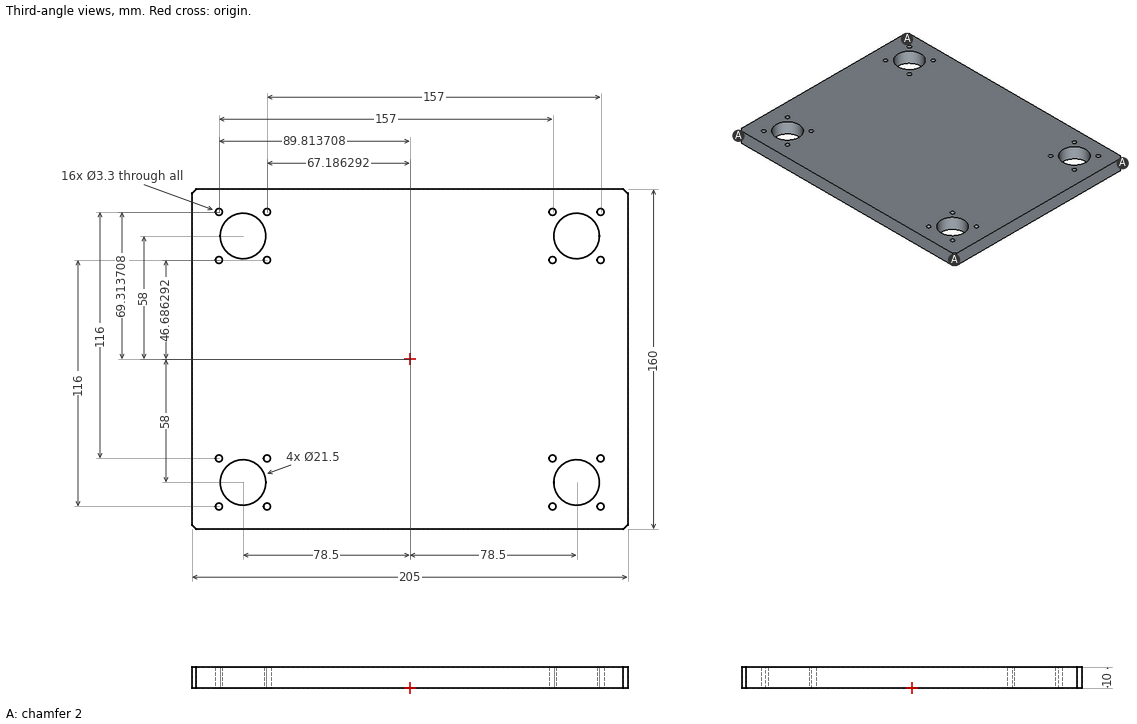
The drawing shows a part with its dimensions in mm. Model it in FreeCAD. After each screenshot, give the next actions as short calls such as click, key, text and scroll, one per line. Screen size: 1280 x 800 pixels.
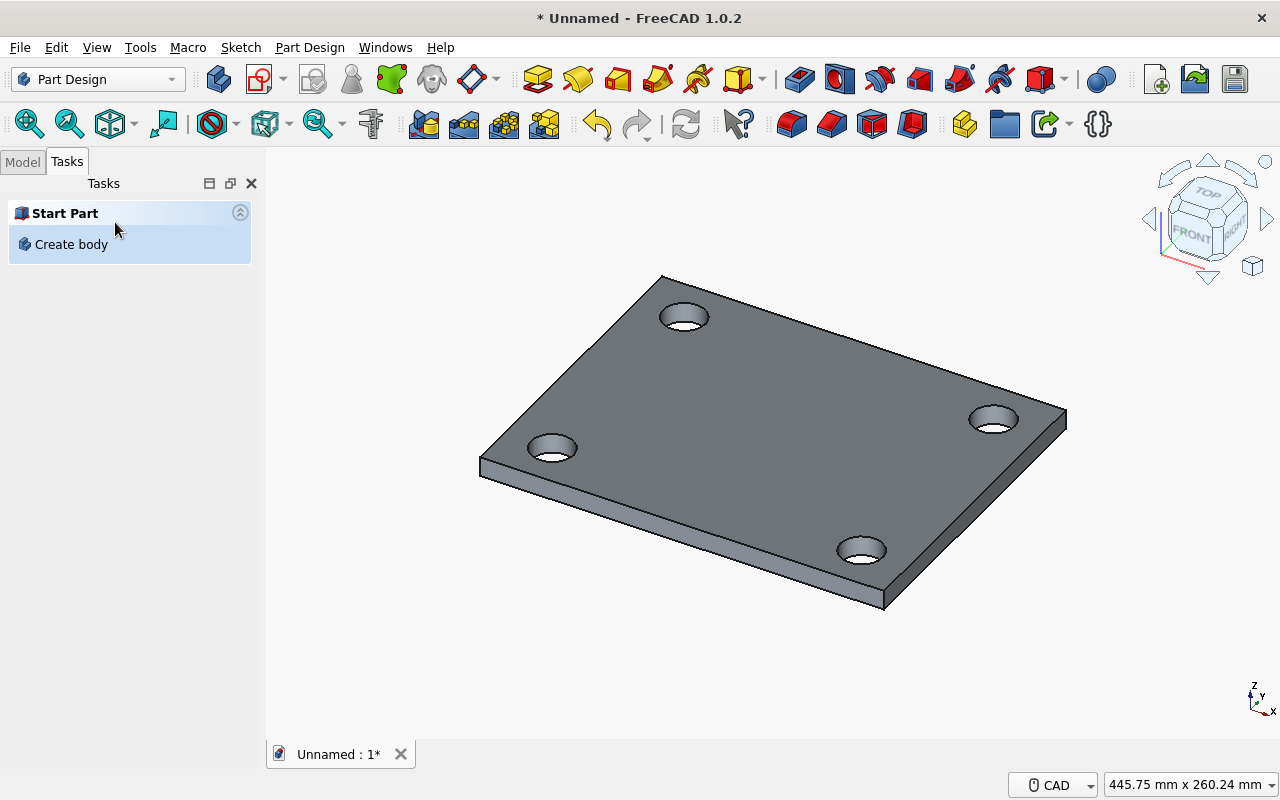
click(773, 433)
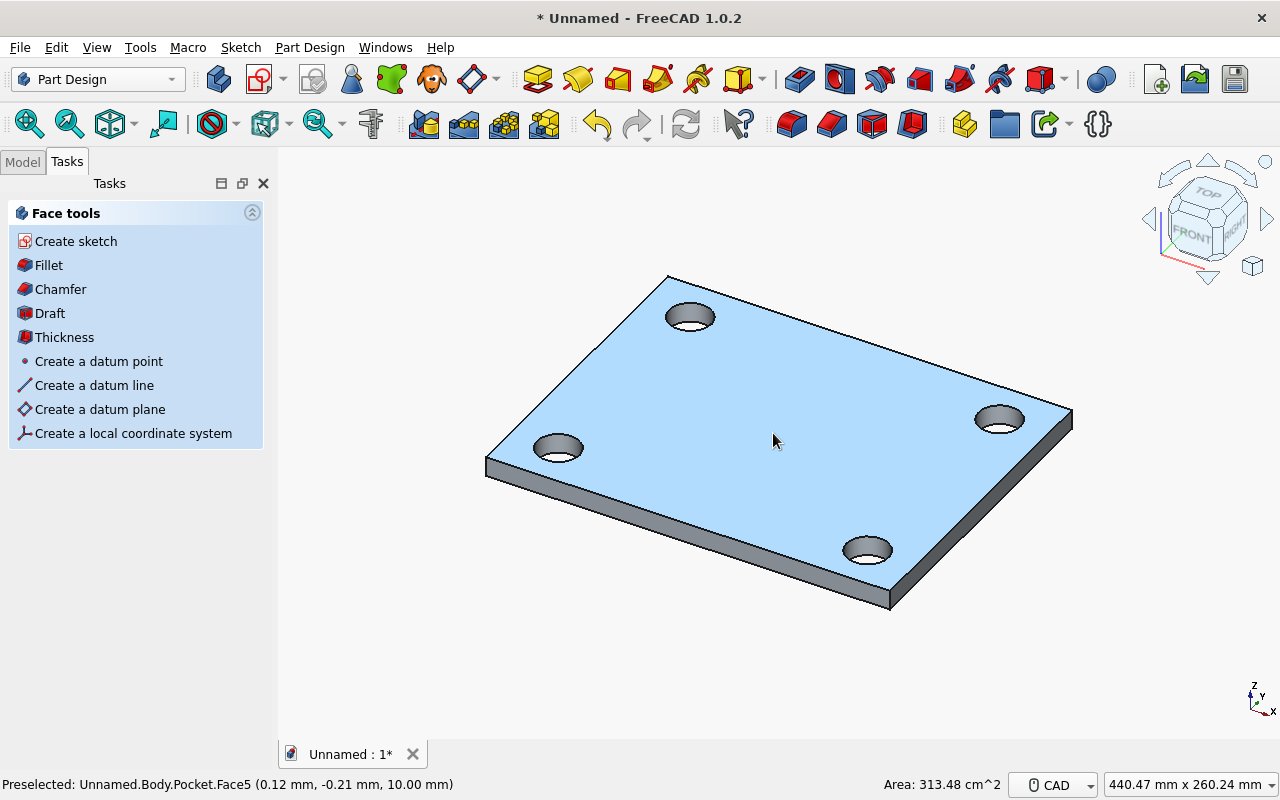
click(260, 80)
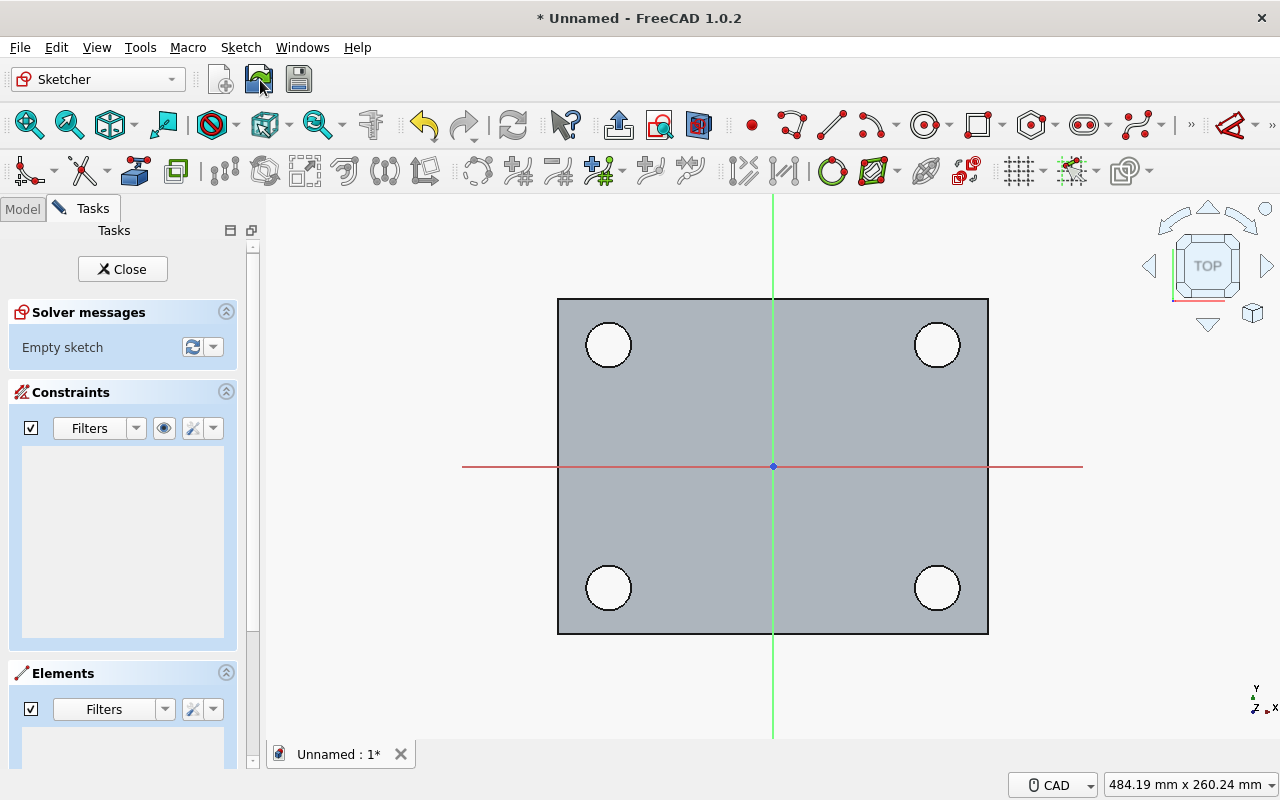
key(g)
key(c)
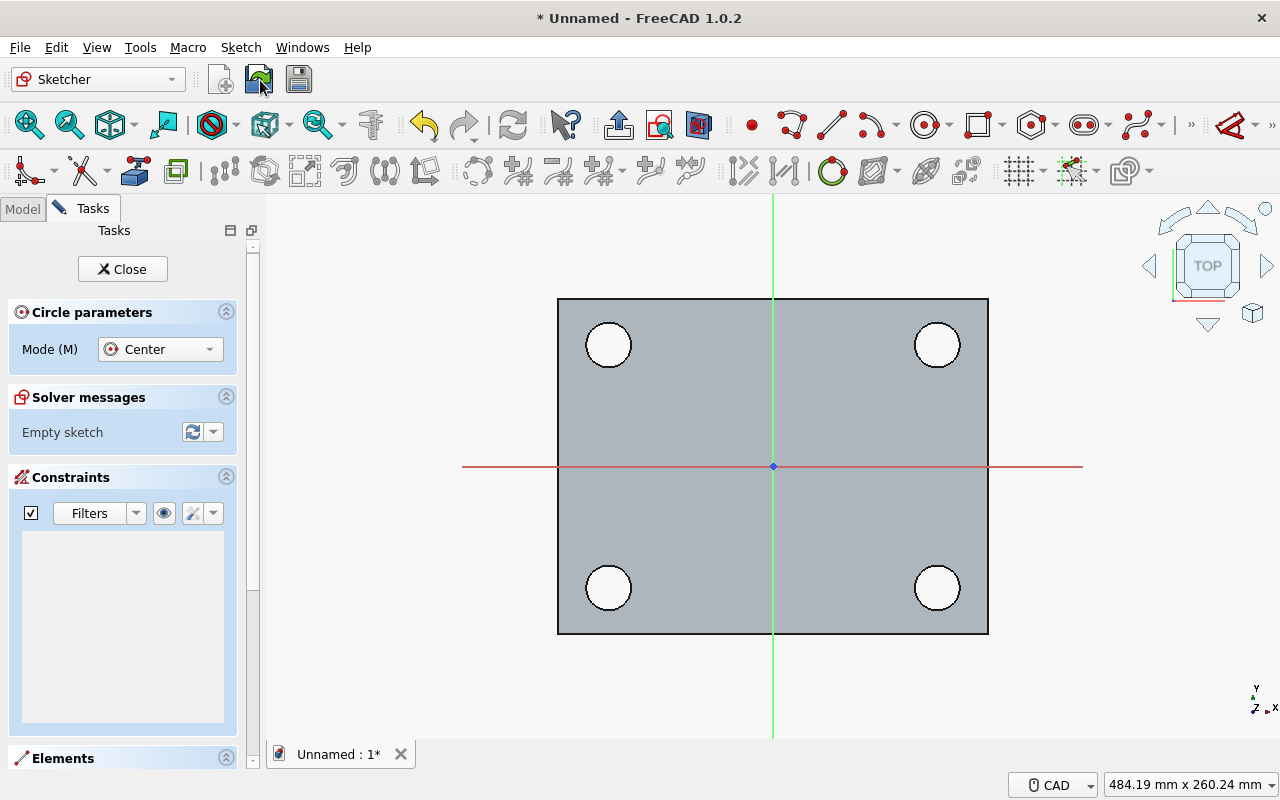
scroll(585, 321, up, 10)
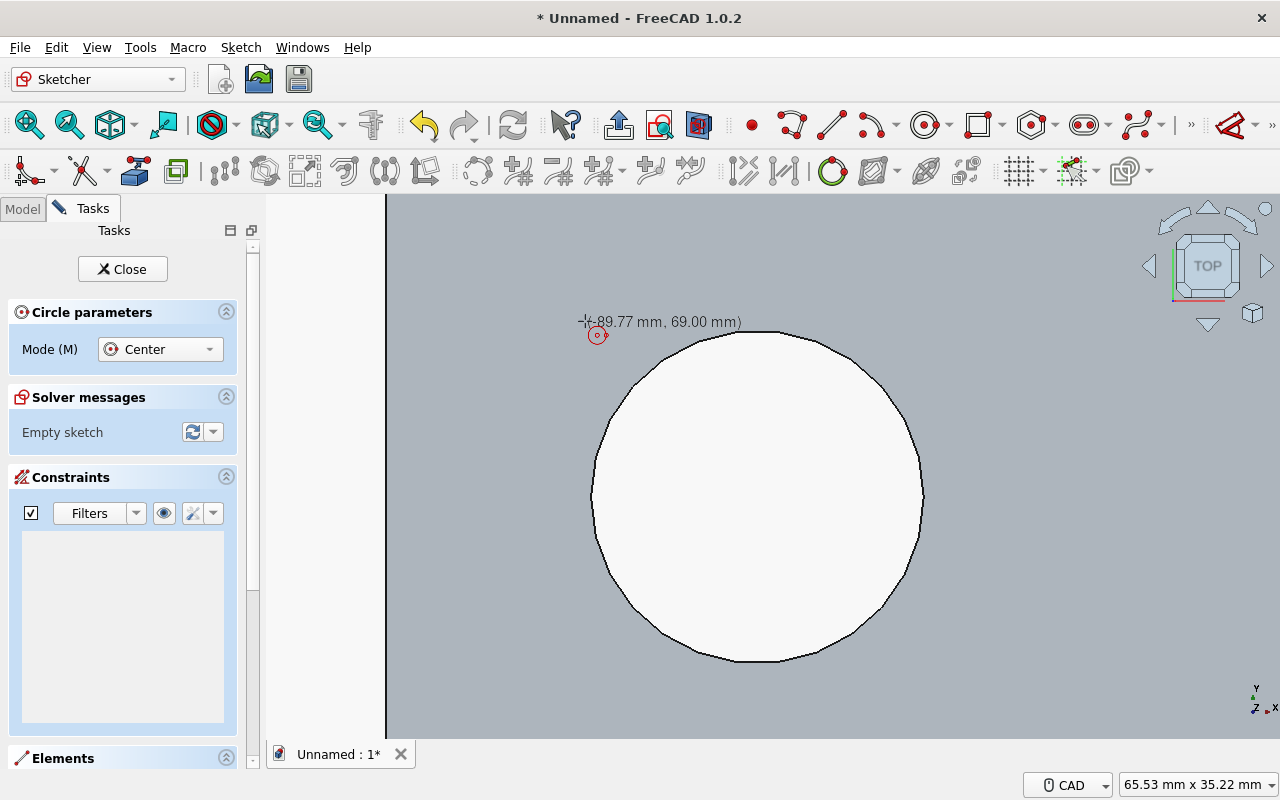
scroll(453, 283, down, 9)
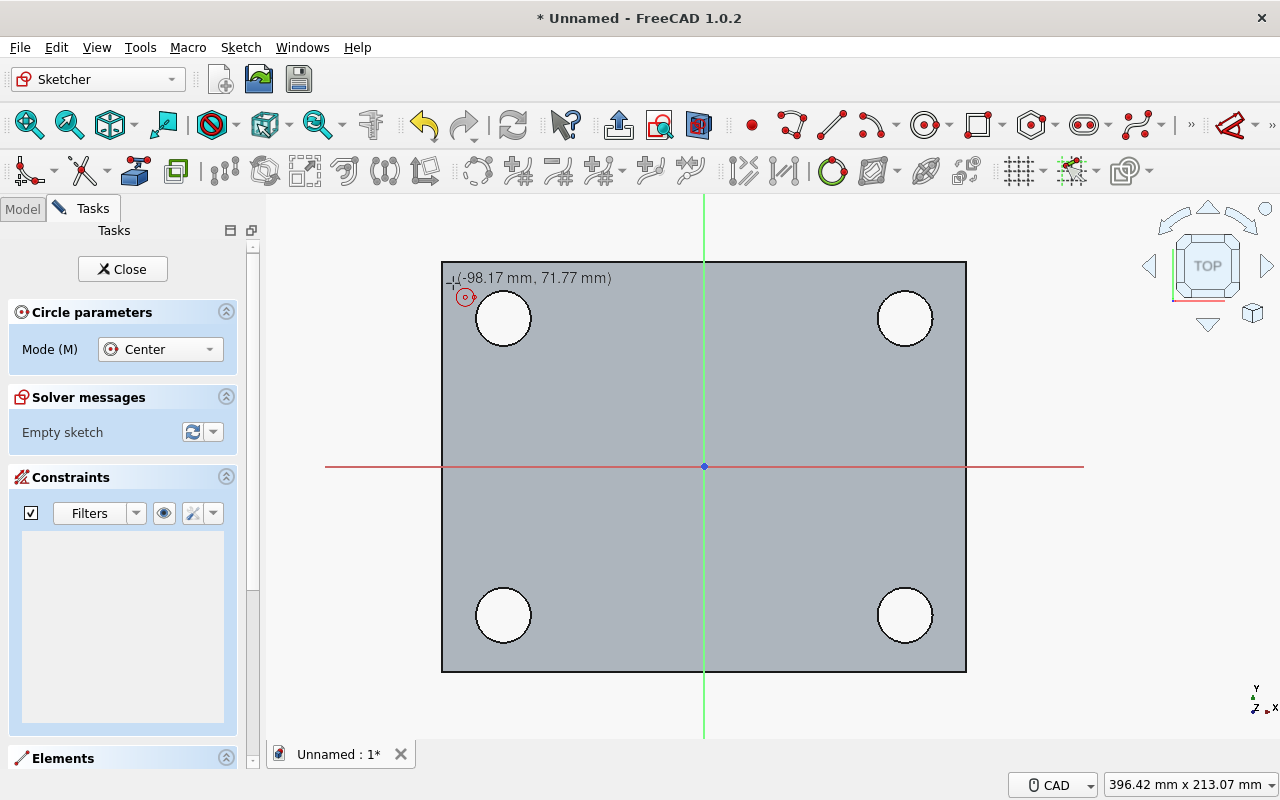
click(475, 290)
move(478, 287)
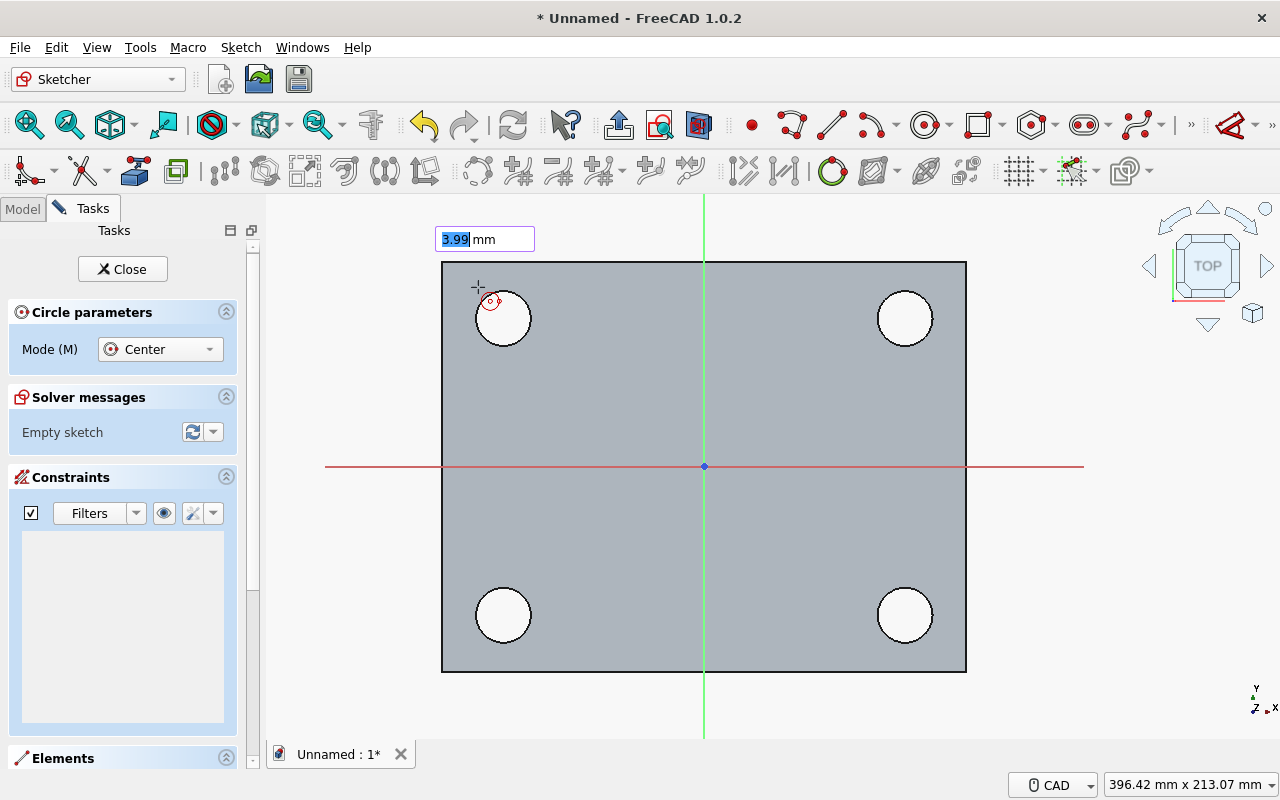
text(3.3)
key(Return)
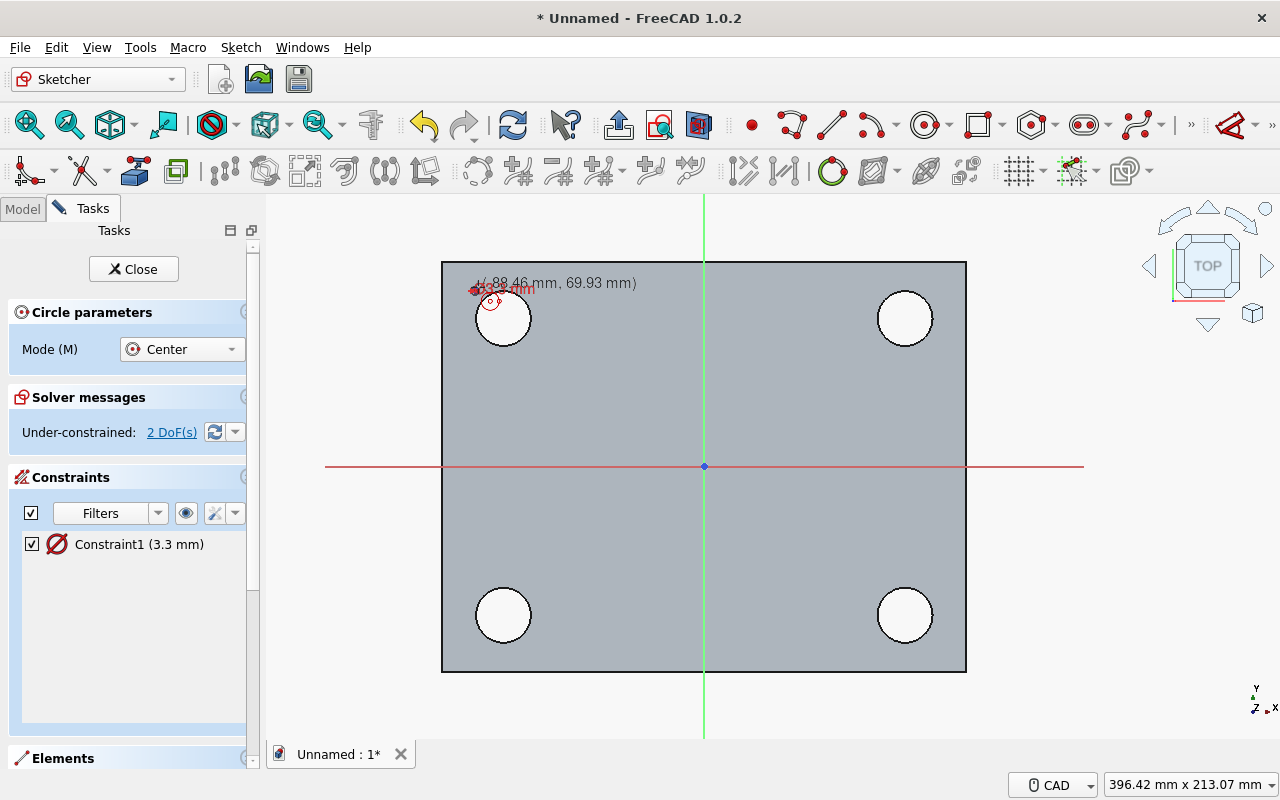
scroll(532, 290, up, 9)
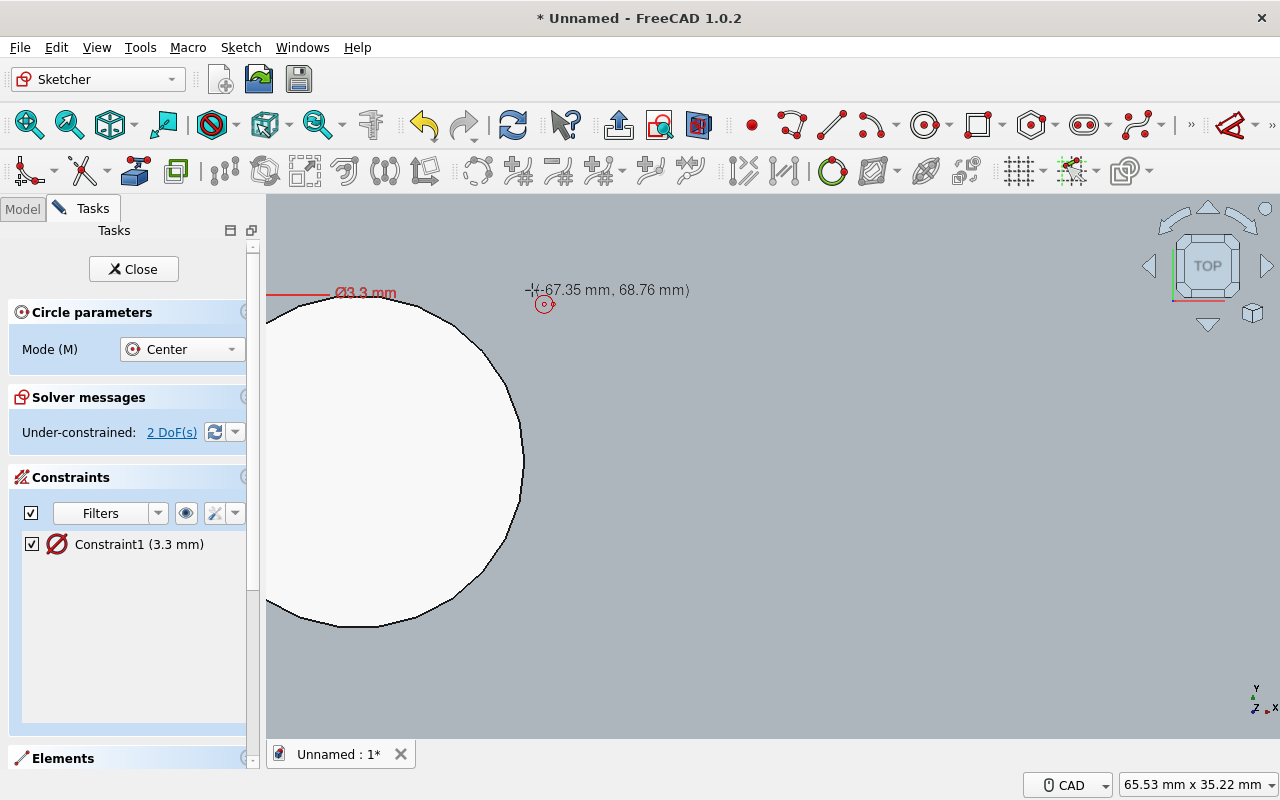
scroll(533, 290, down, 9)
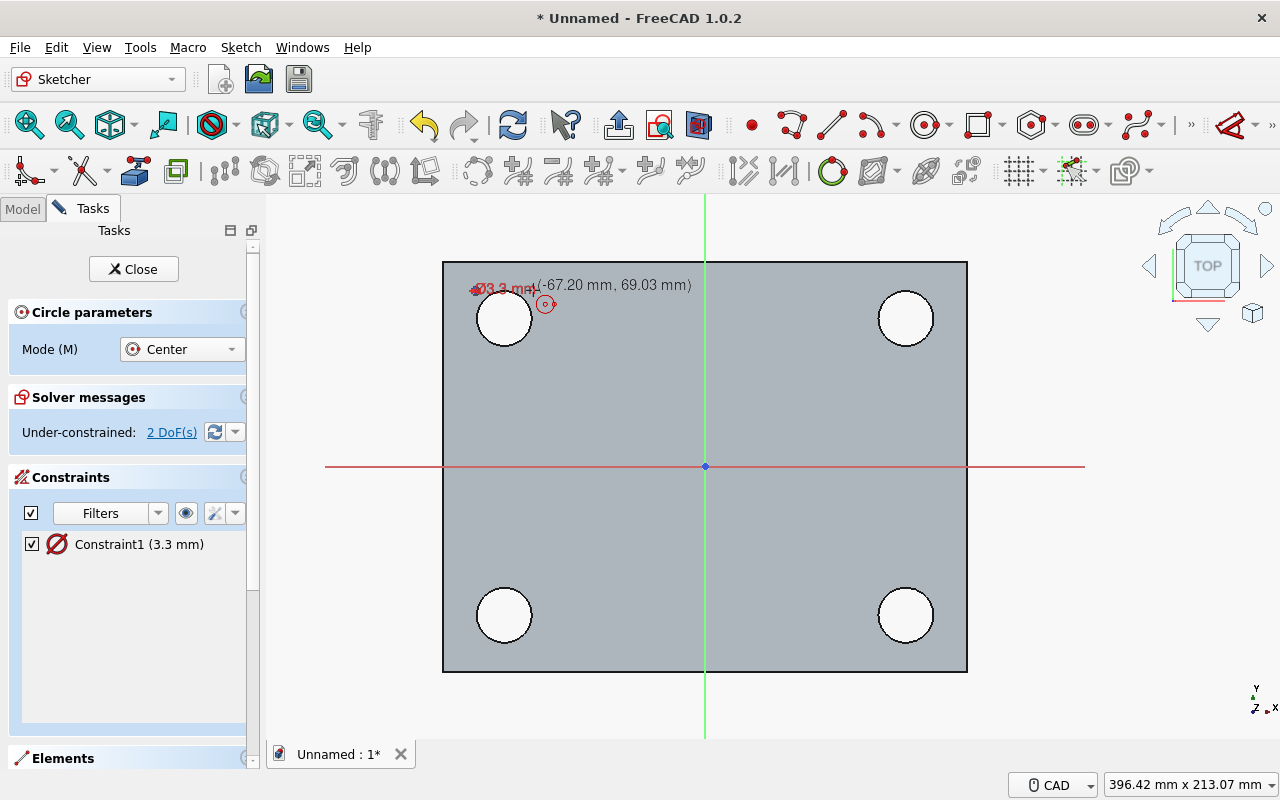
click(533, 290)
move(536, 287)